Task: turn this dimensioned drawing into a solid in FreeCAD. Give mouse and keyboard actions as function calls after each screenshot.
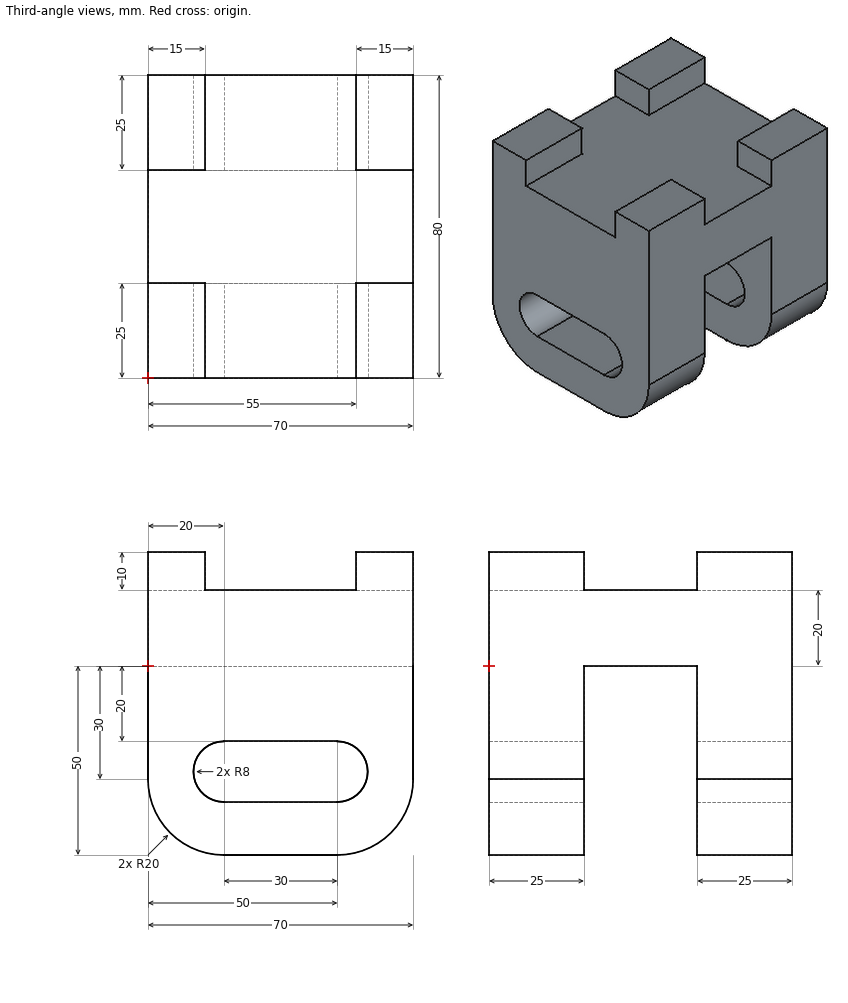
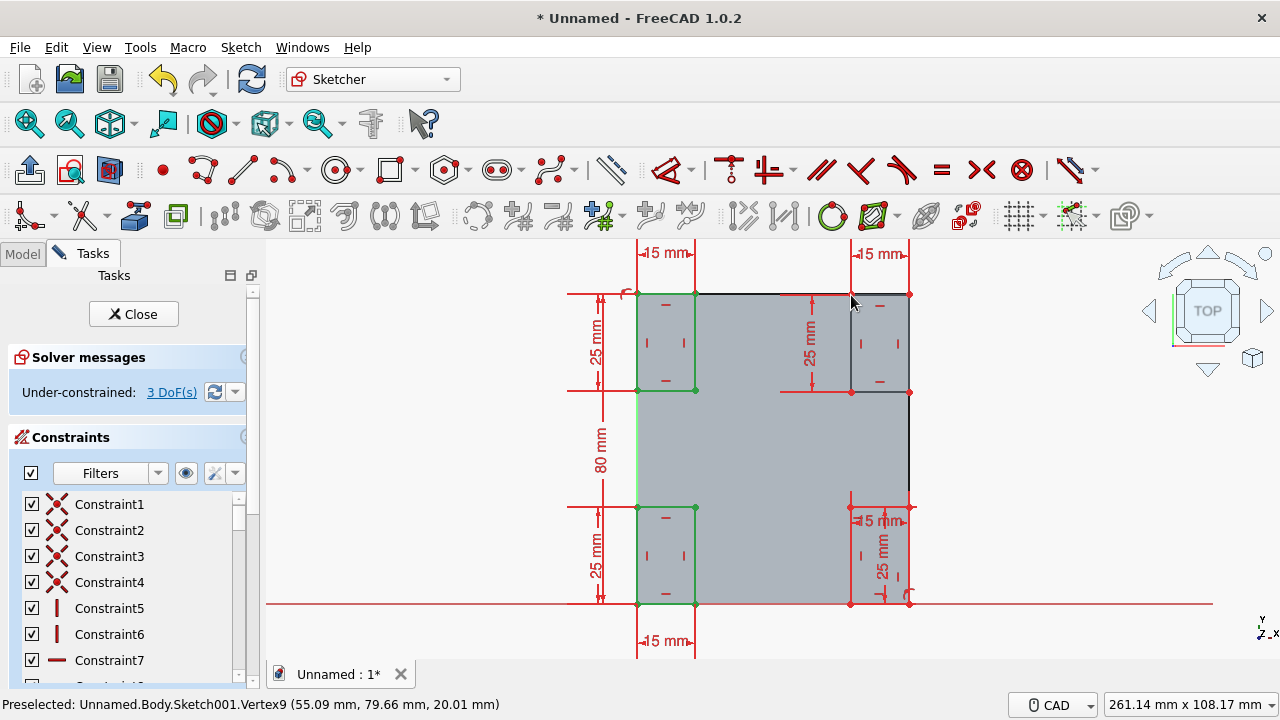
click(851, 295)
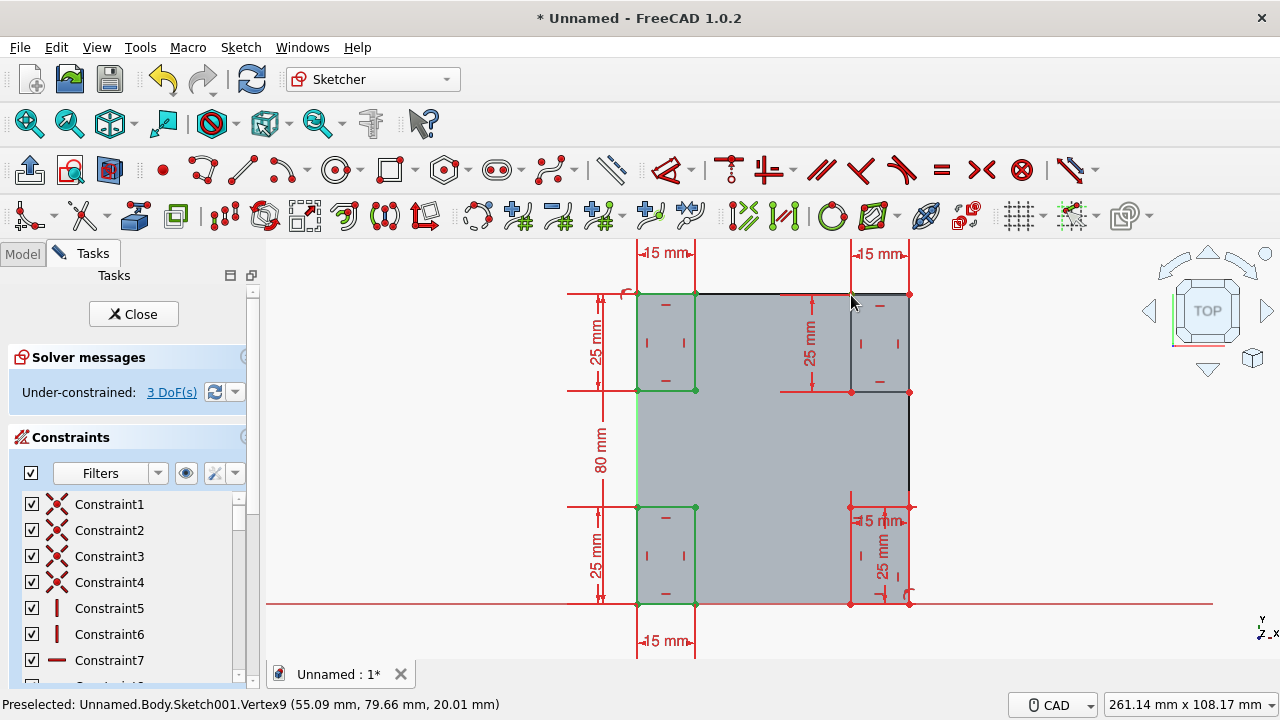
click(694, 170)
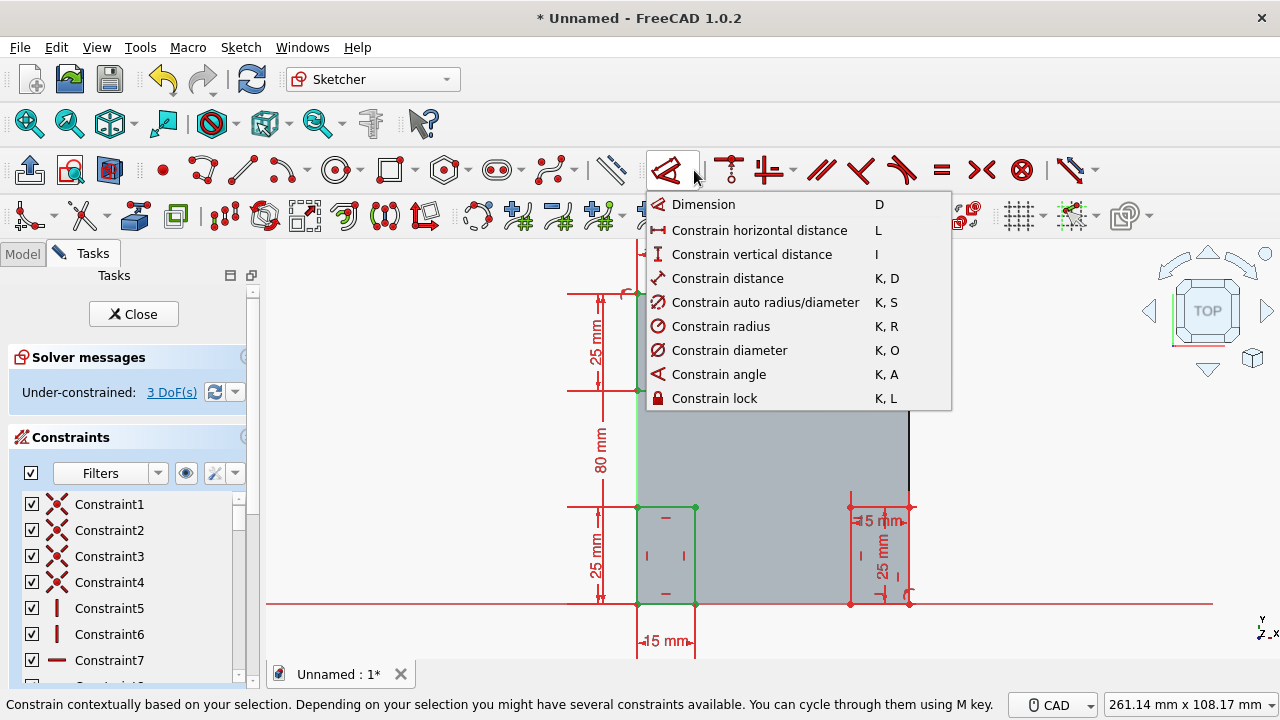
click(799, 230)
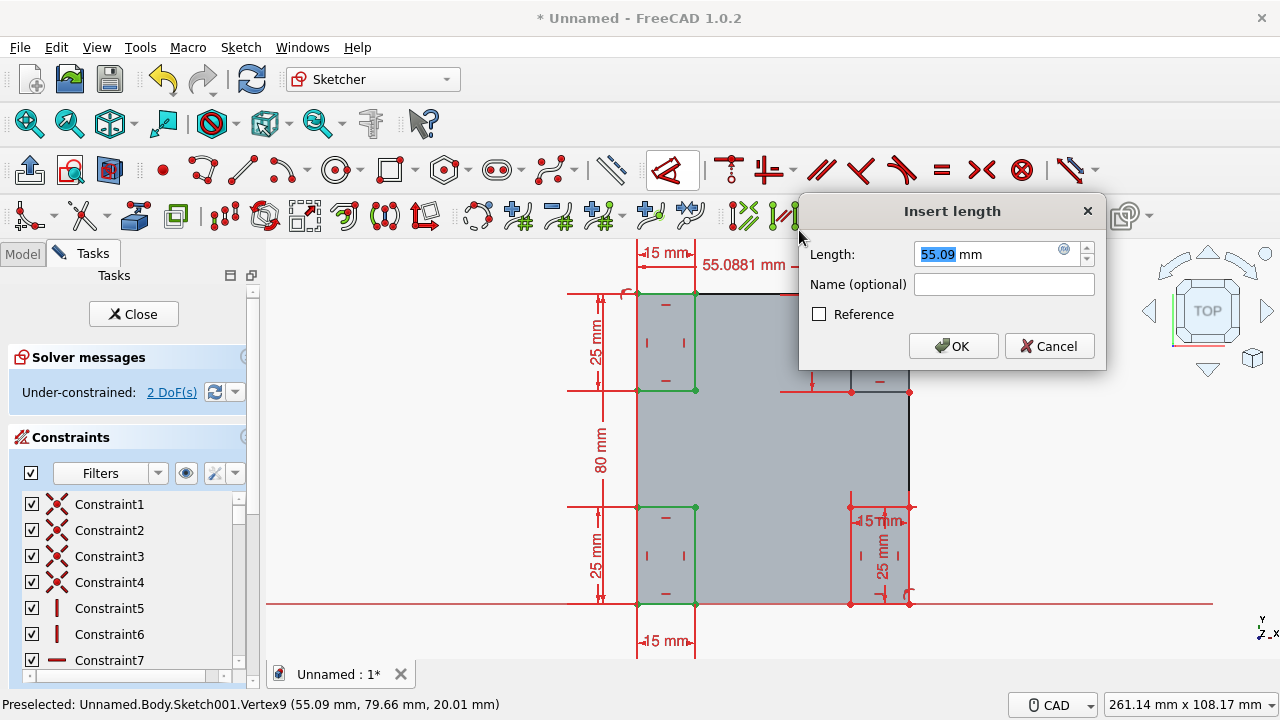
text(55)
key(Return)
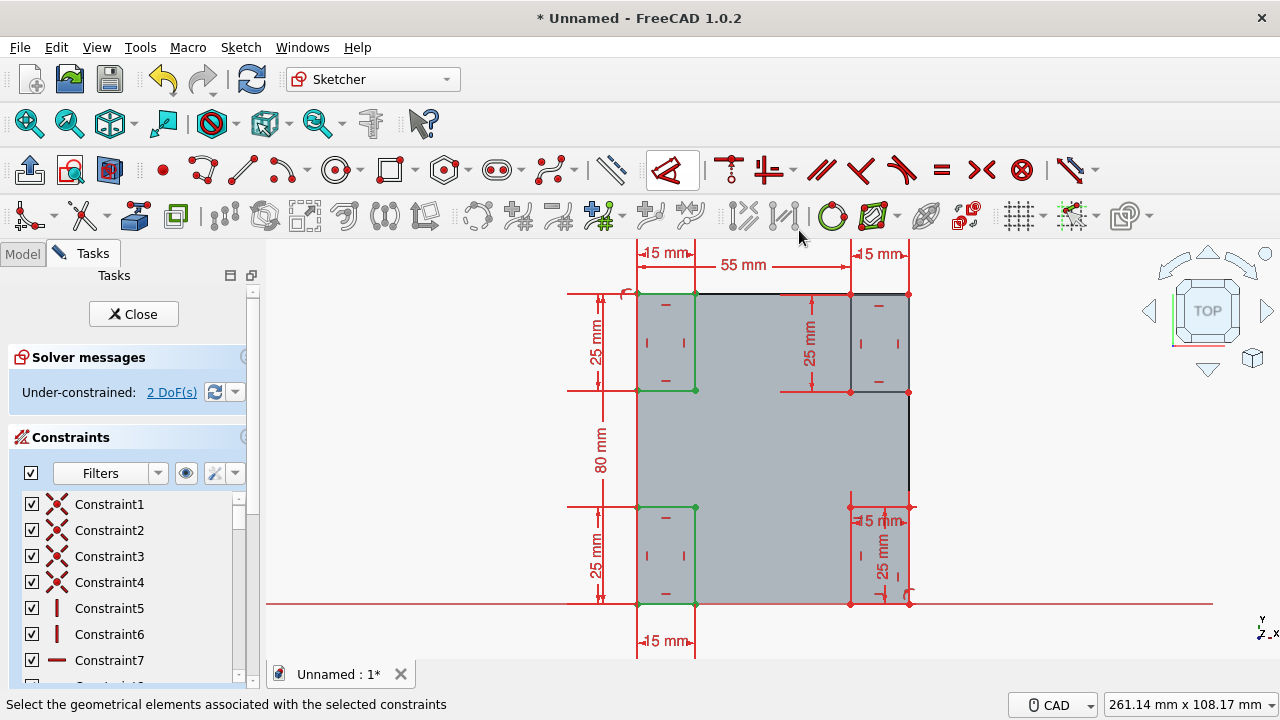
click(851, 295)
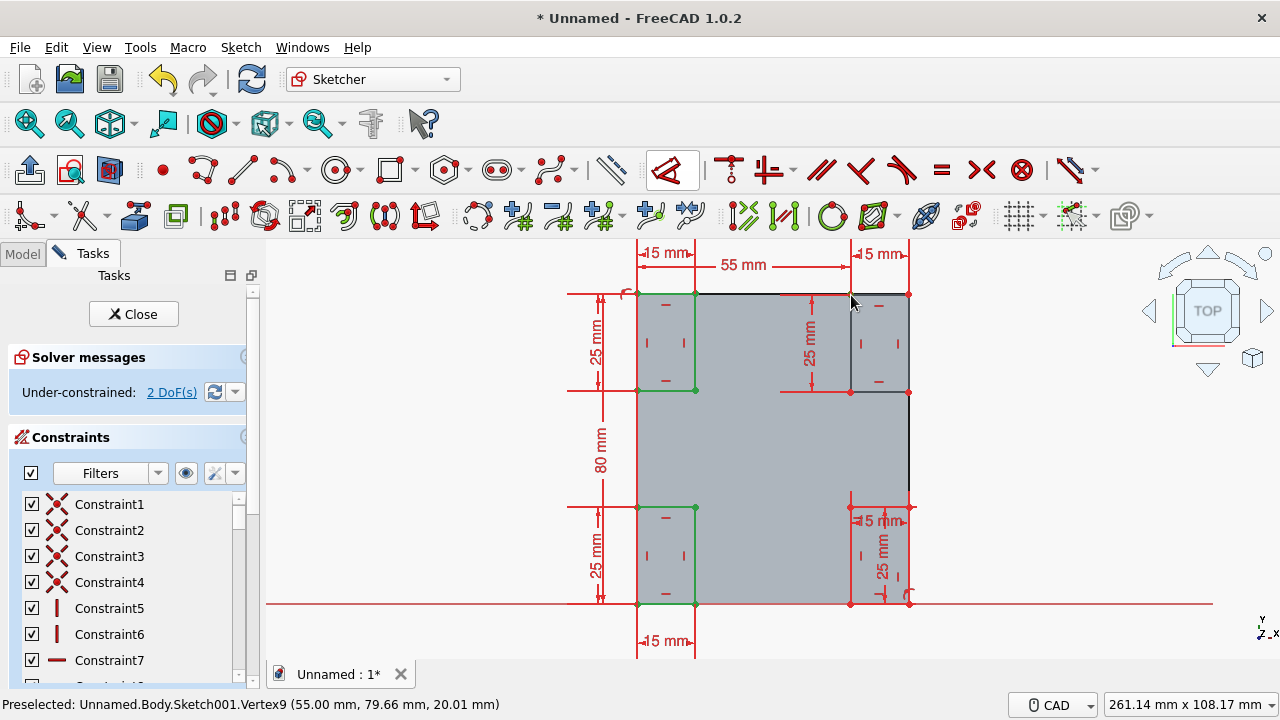
key(i)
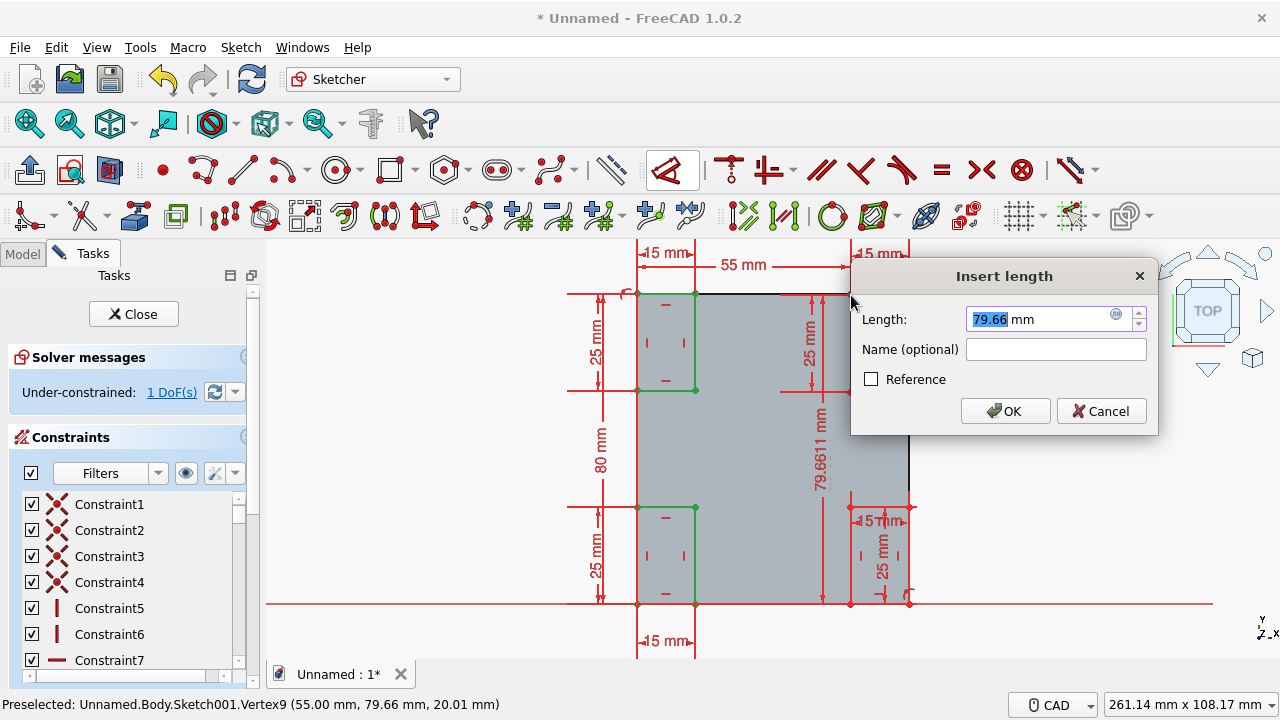
text(80)
key(Return)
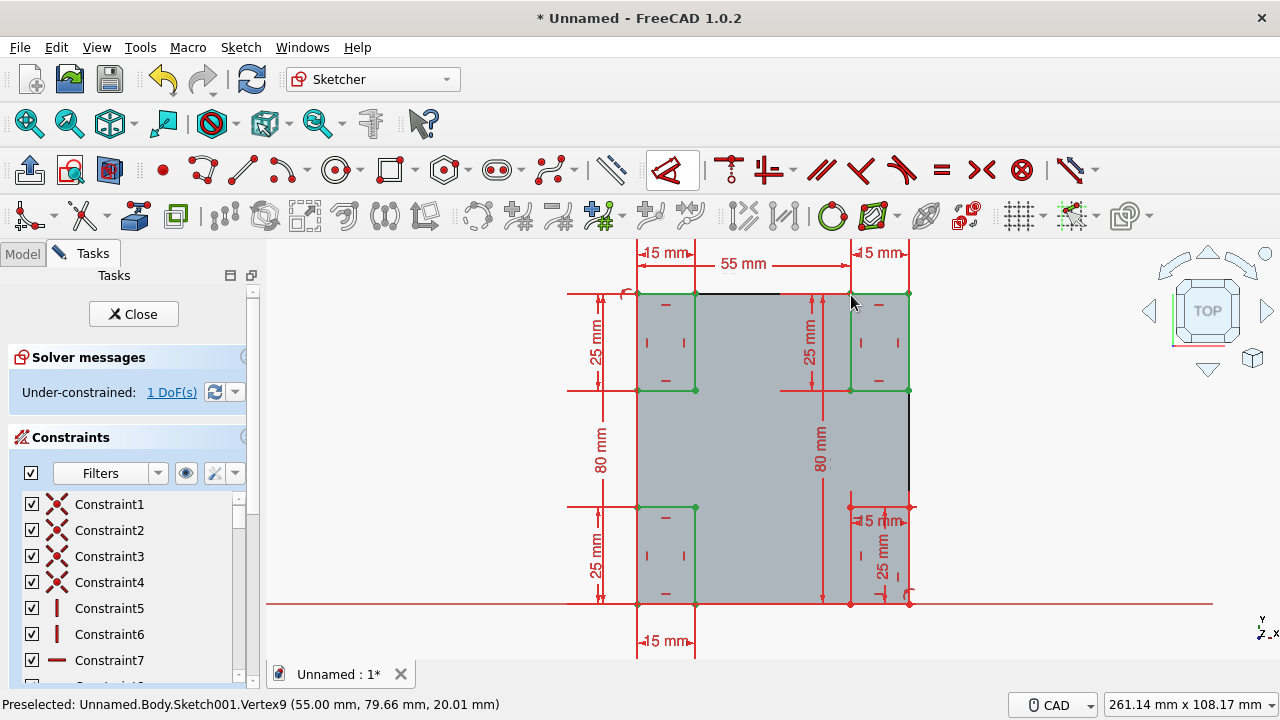
click(851, 507)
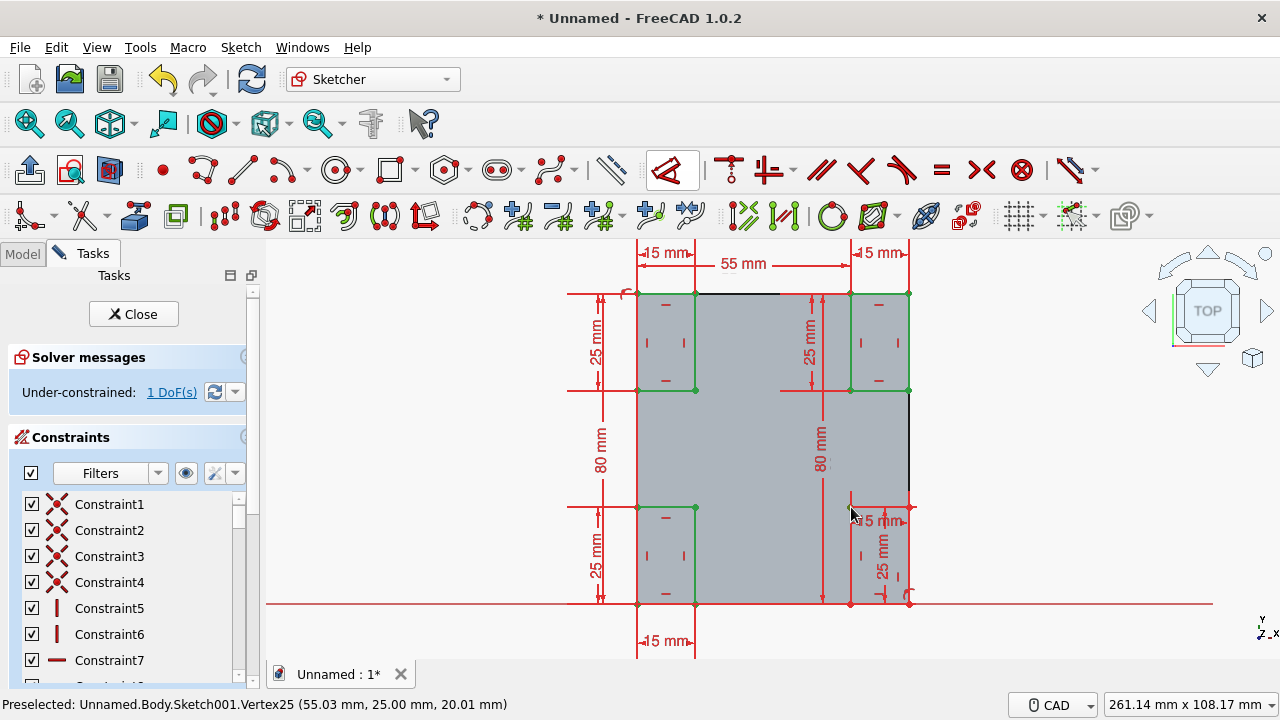
click(694, 170)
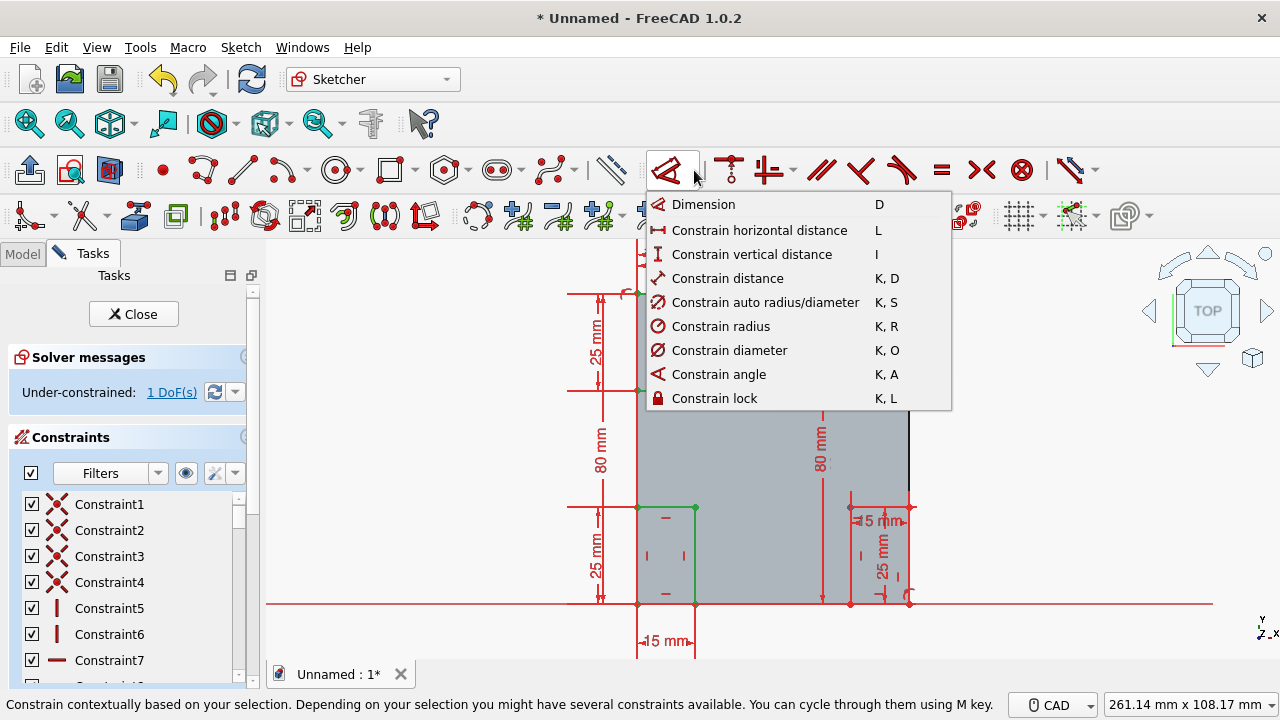
click(799, 230)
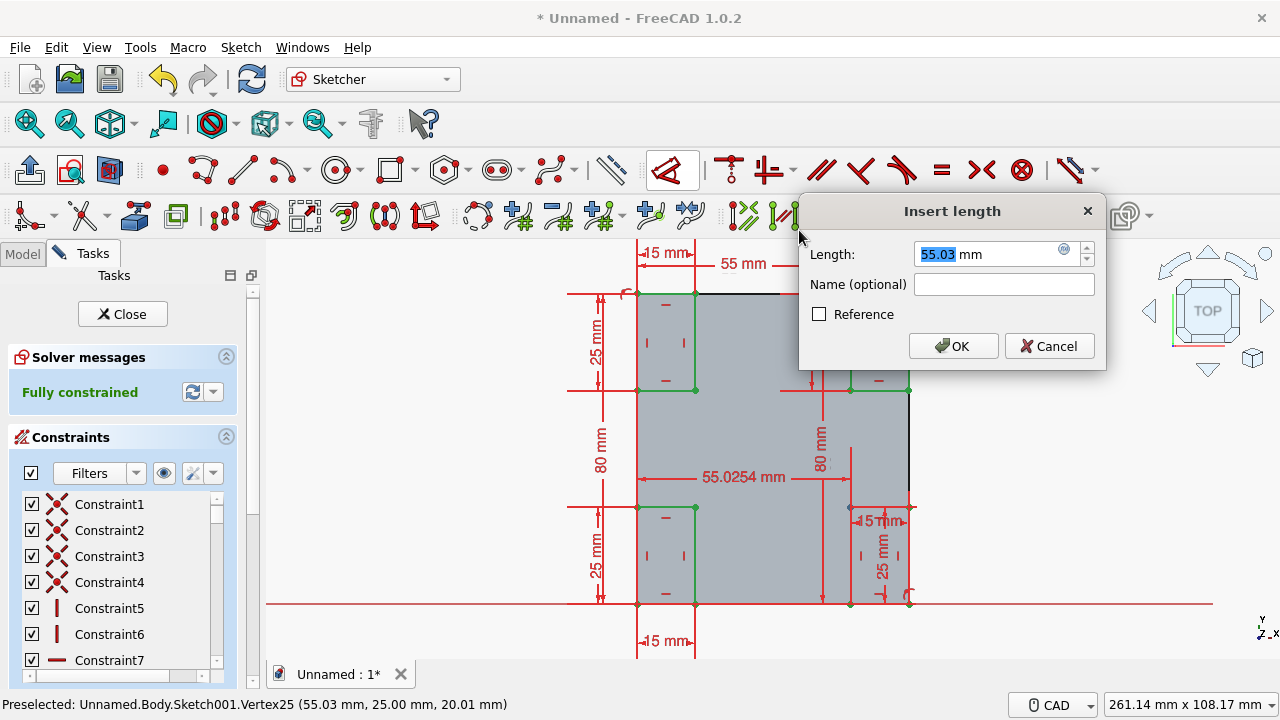
text(55)
key(Return)